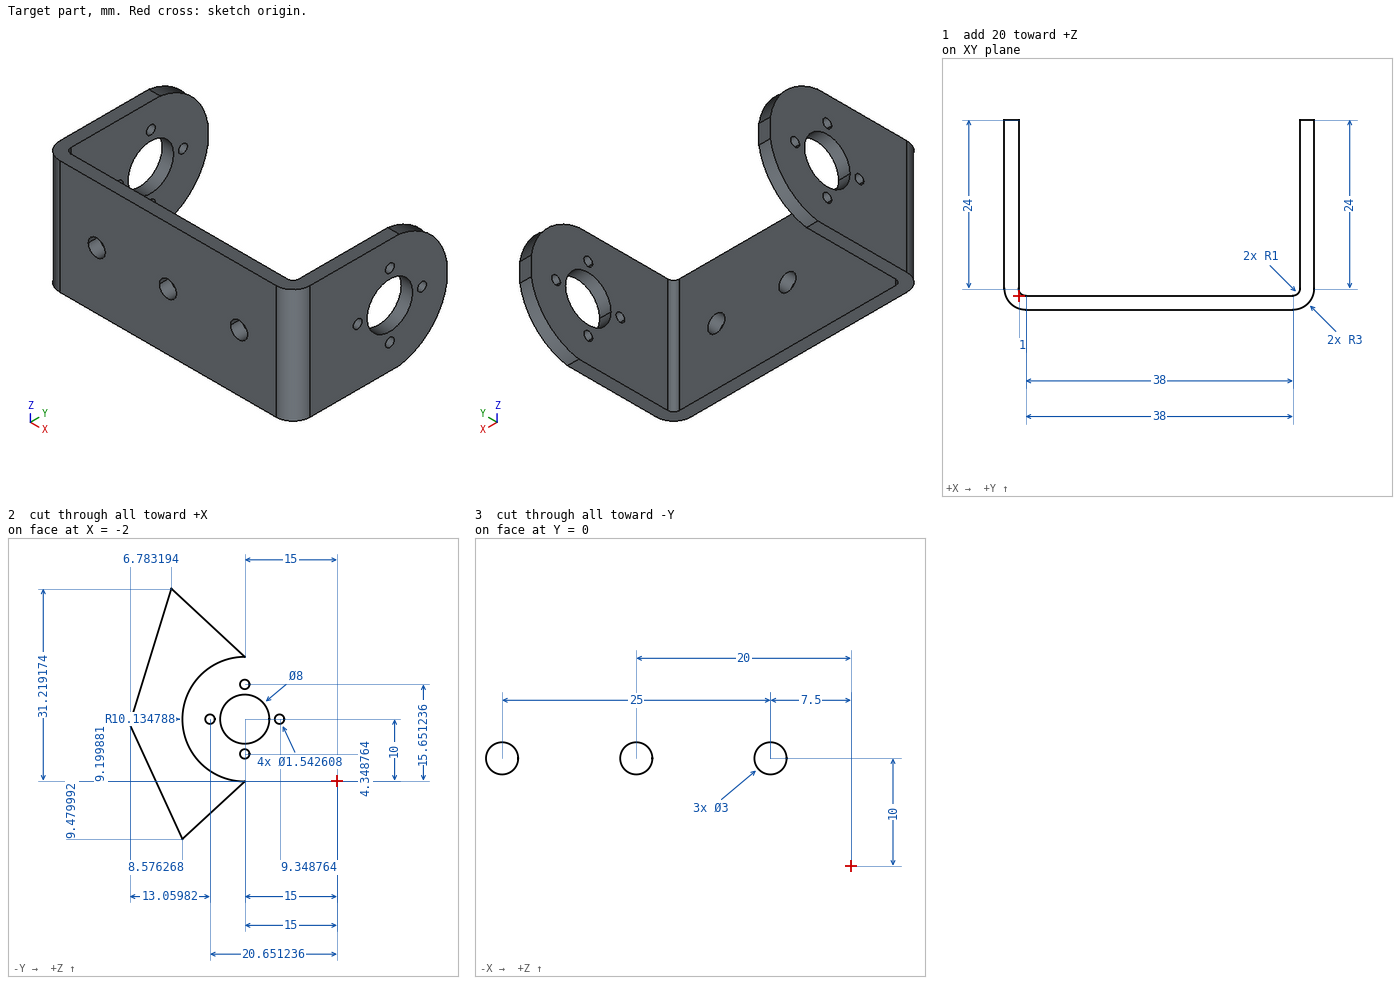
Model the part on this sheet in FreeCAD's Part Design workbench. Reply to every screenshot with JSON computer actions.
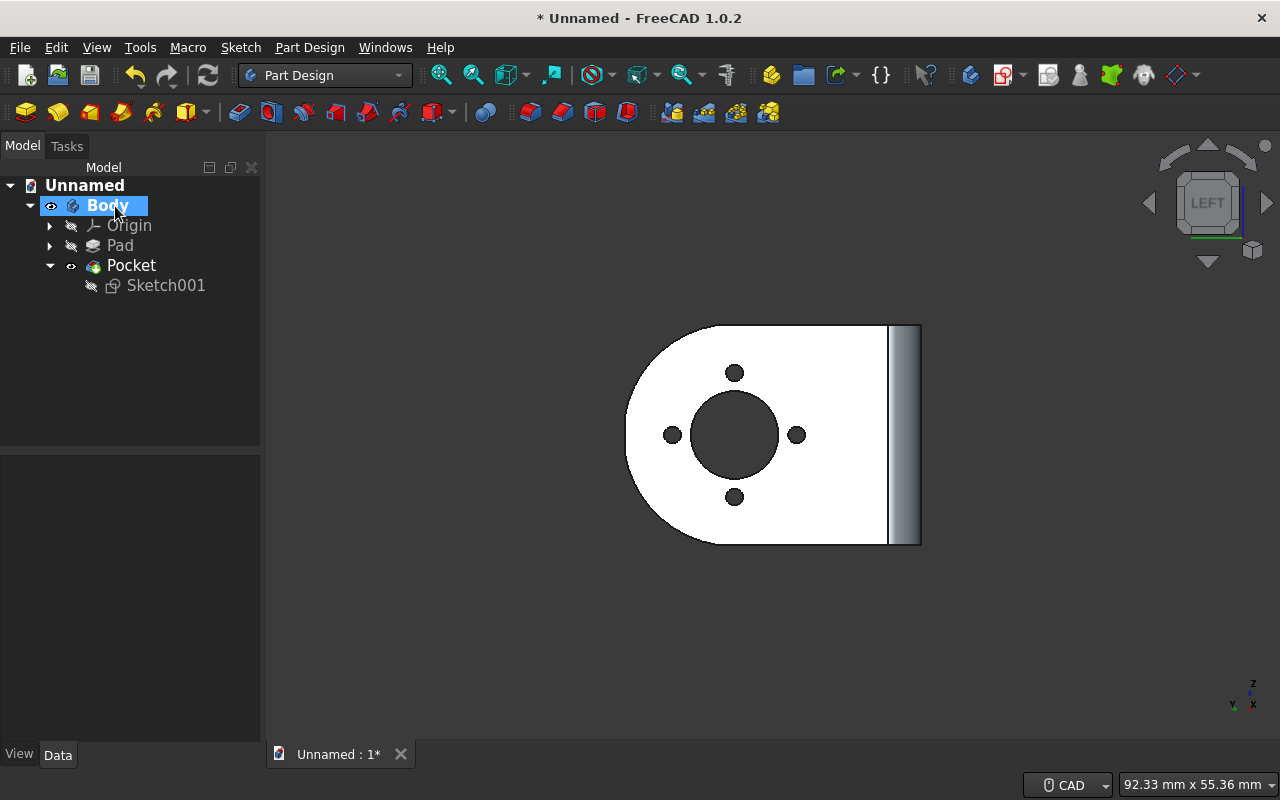
{"action": "left_click", "coordinate": [442, 76]}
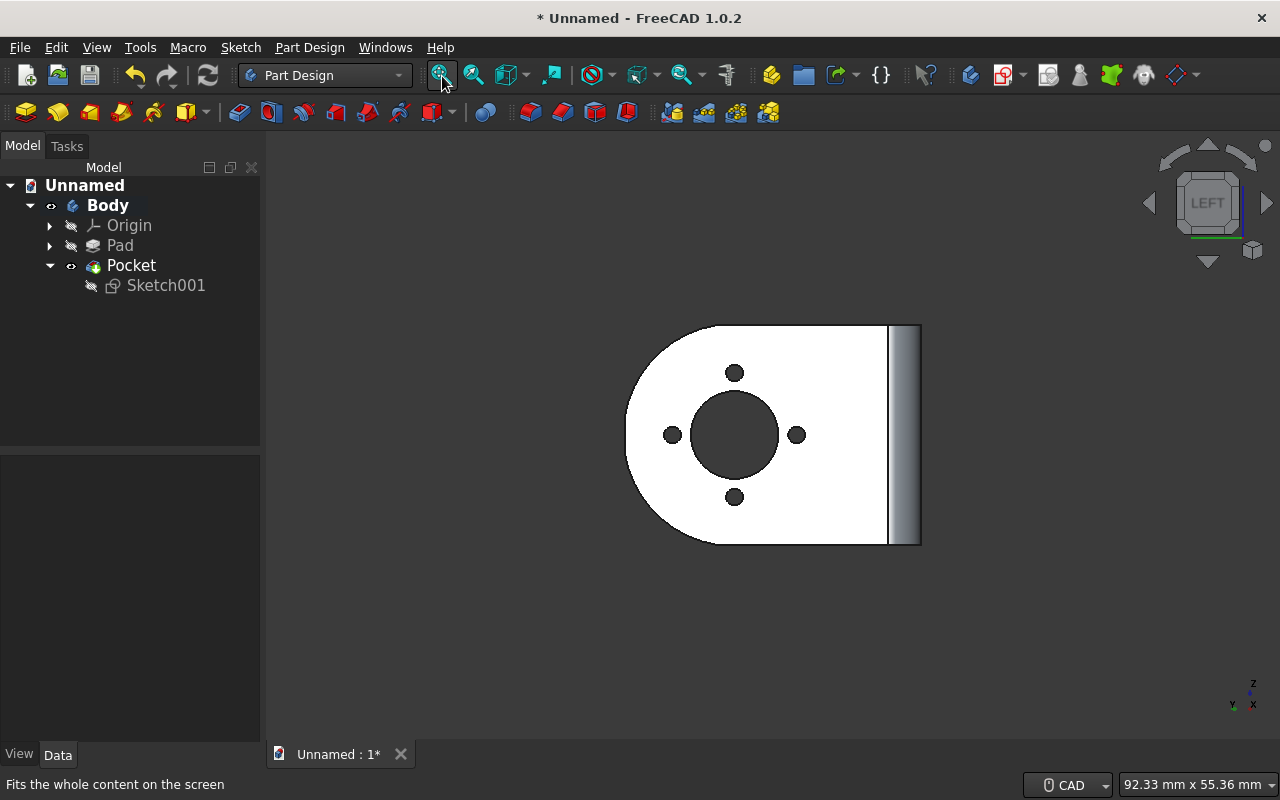
{"action": "key", "text": "4"}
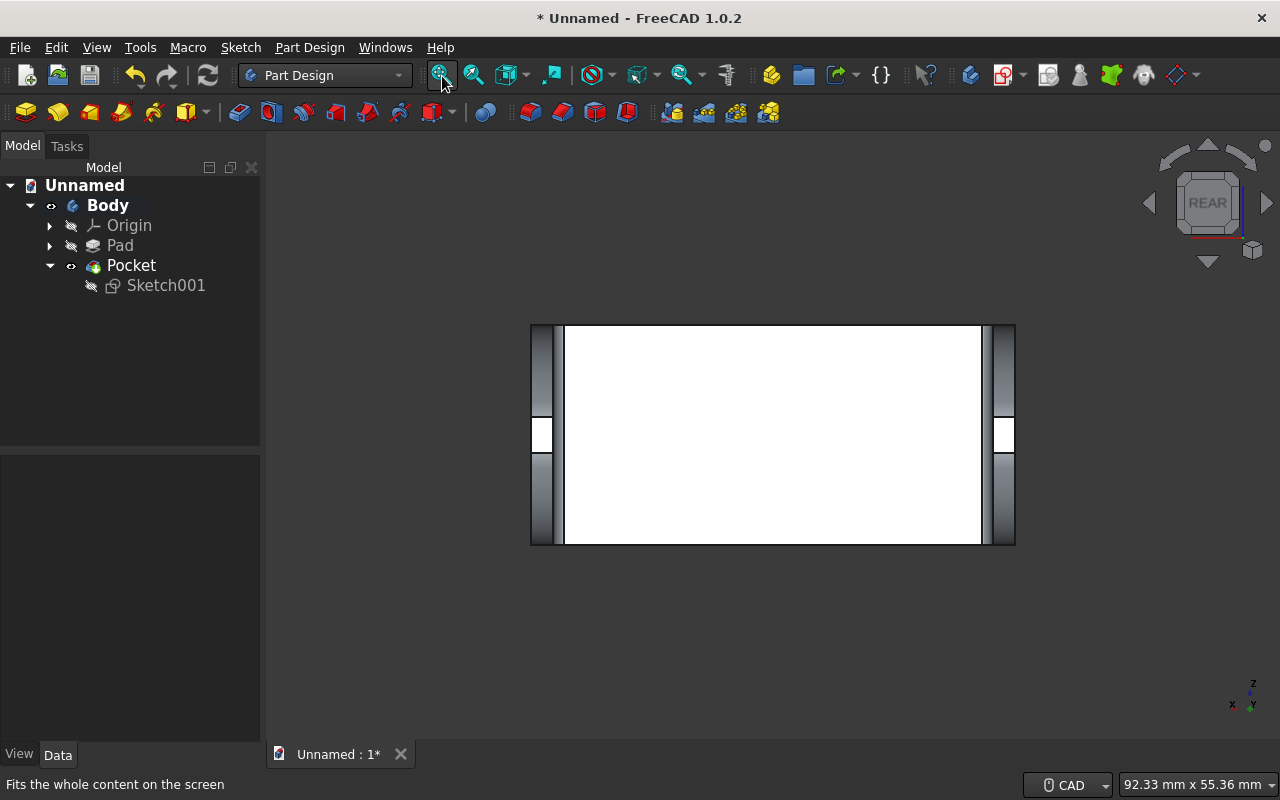
{"action": "left_click", "coordinate": [713, 434]}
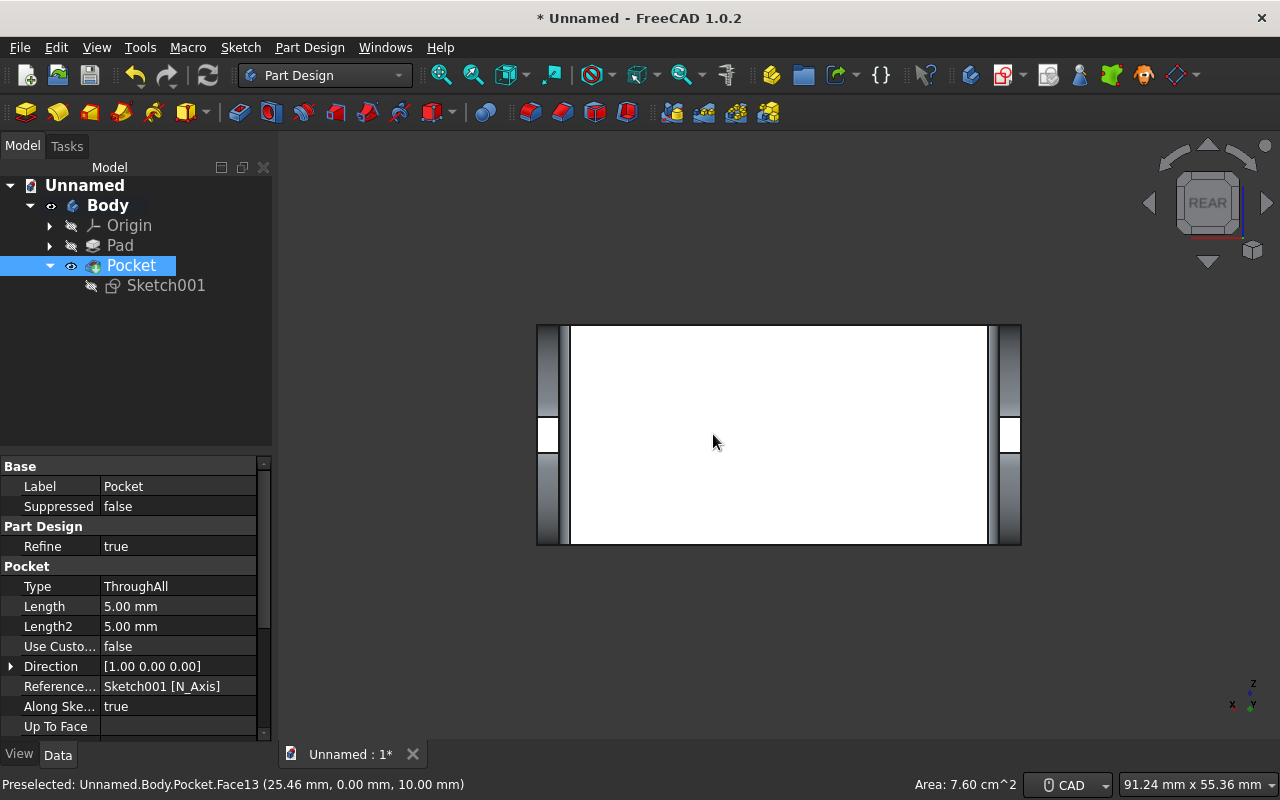
{"action": "left_click", "coordinate": [1004, 76]}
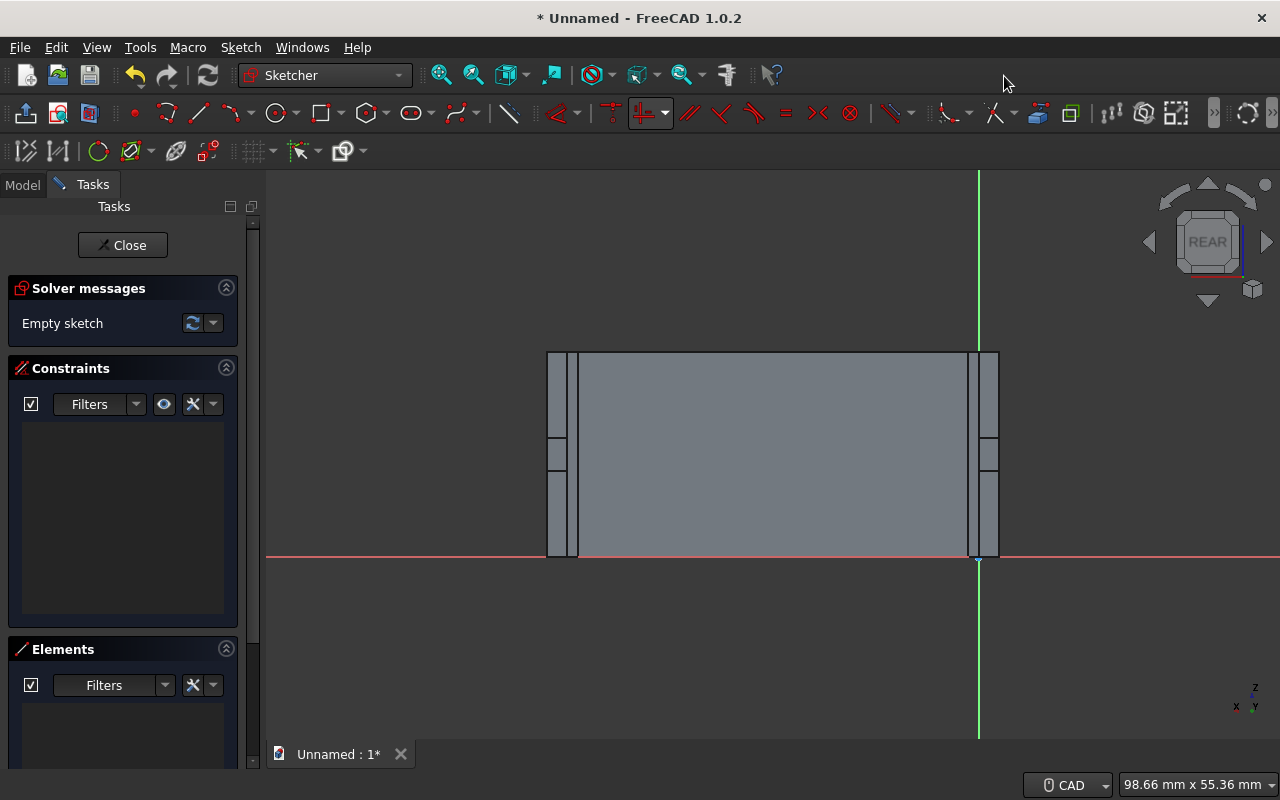
{"action": "left_click", "coordinate": [90, 114]}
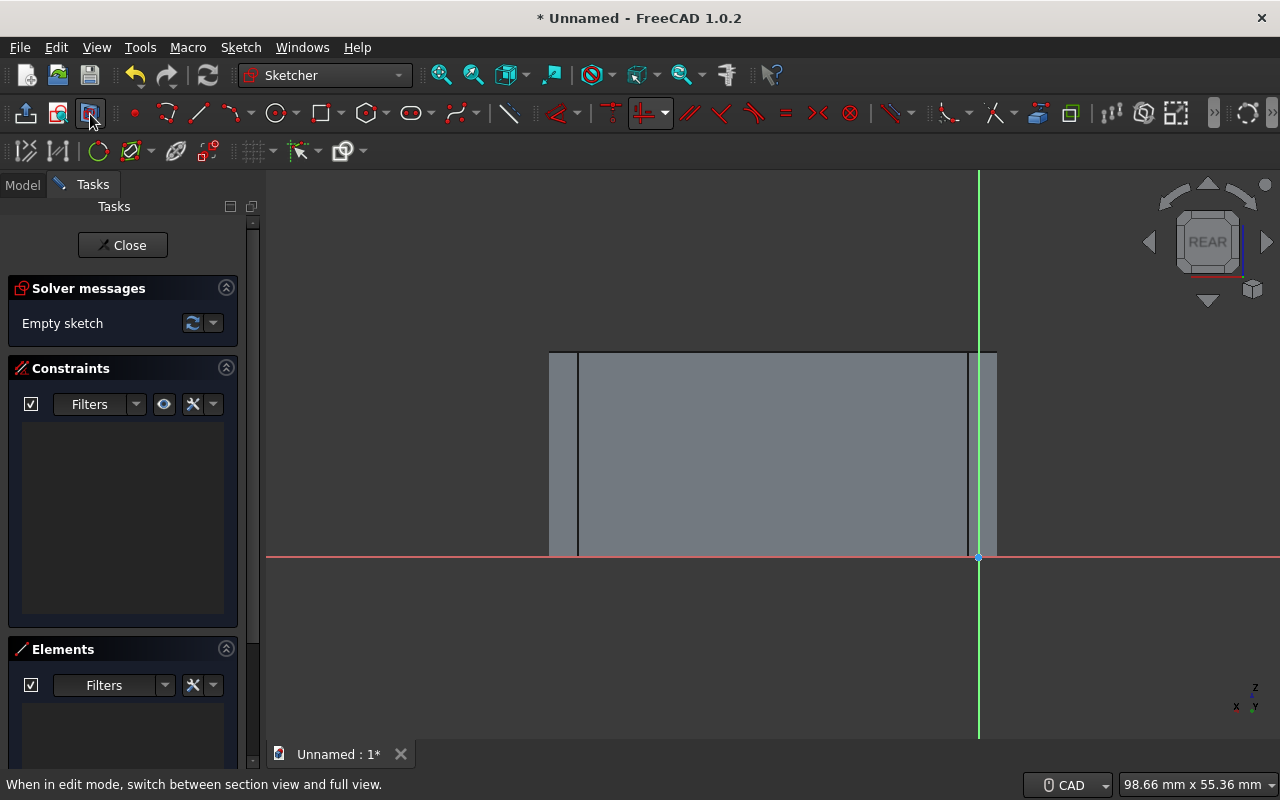
{"action": "scroll", "coordinate": [925, 551], "scroll_direction": "up", "scroll_amount": 3}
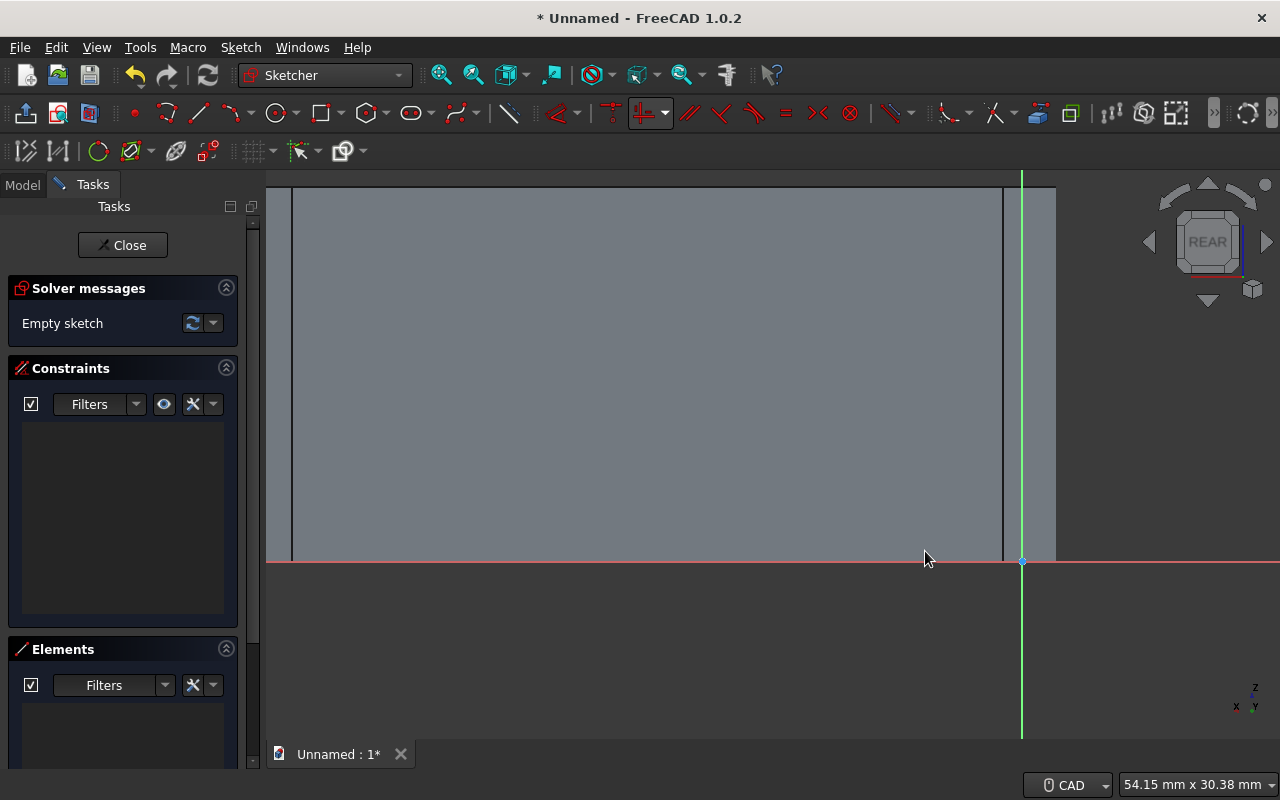
{"action": "left_click", "coordinate": [276, 114]}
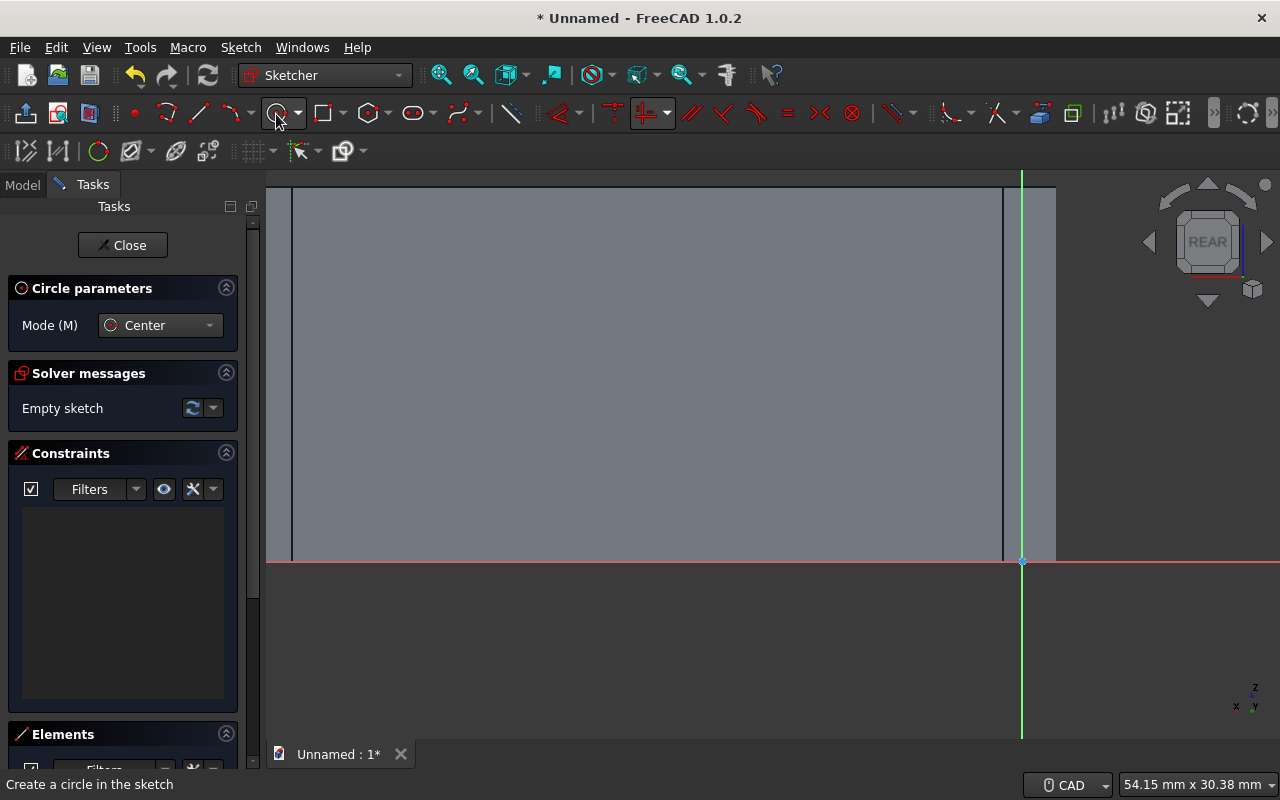
{"action": "left_click", "coordinate": [882, 375]}
{"action": "mouse_move", "coordinate": [901, 355]}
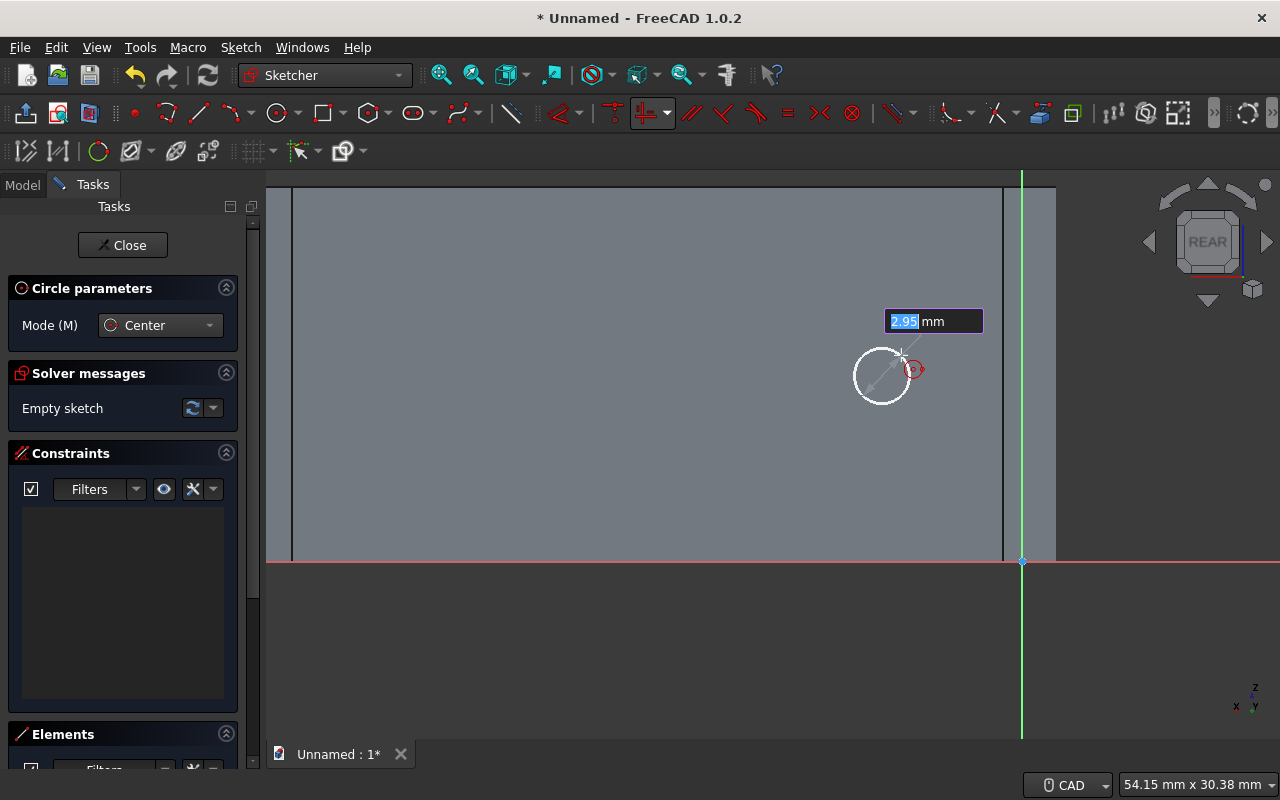
{"action": "type", "text": "3"}
{"action": "key", "text": "Return"}